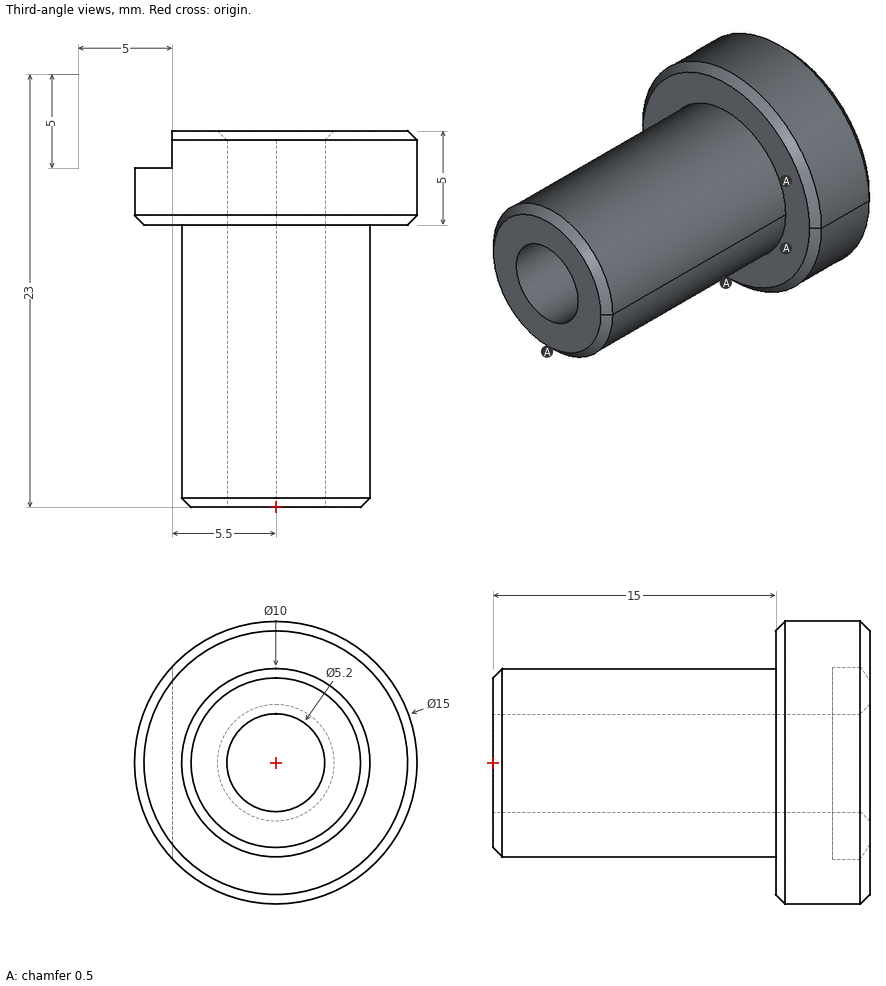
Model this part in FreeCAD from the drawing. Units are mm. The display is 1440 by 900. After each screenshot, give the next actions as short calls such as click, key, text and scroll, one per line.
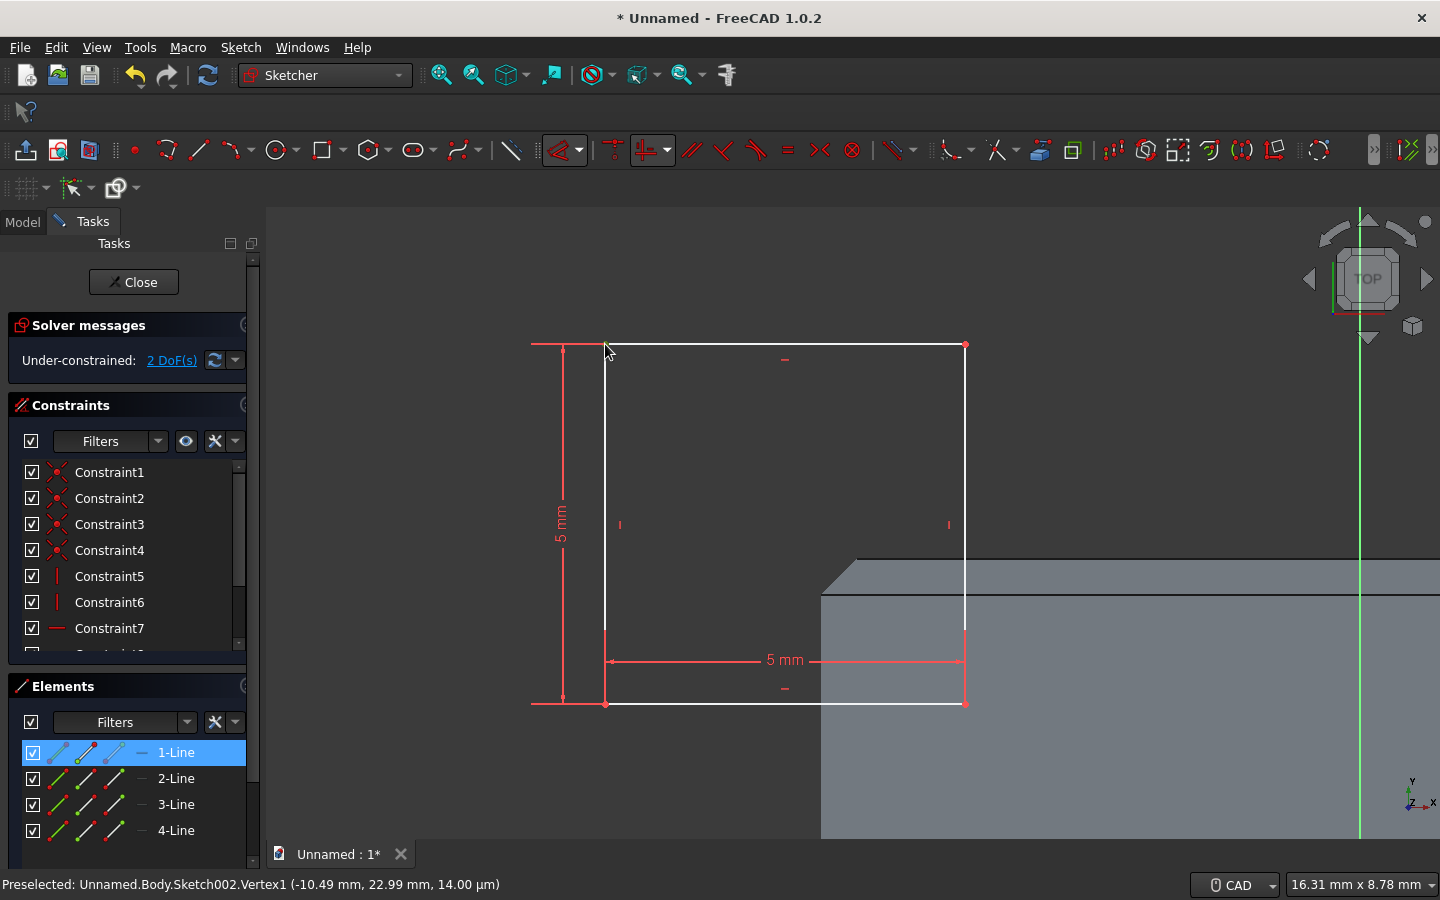
click(582, 150)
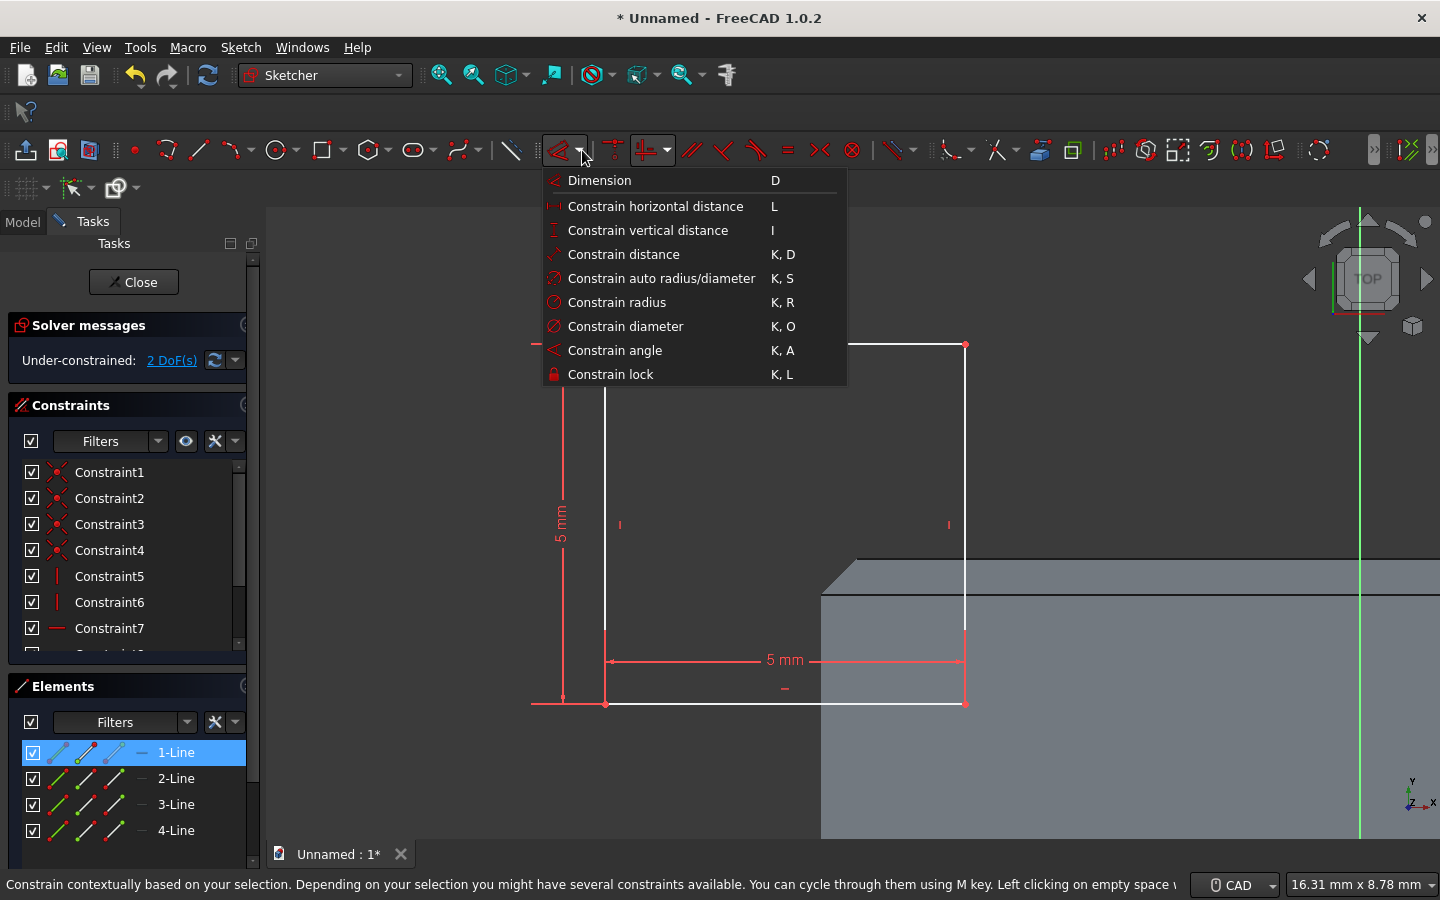
click(695, 230)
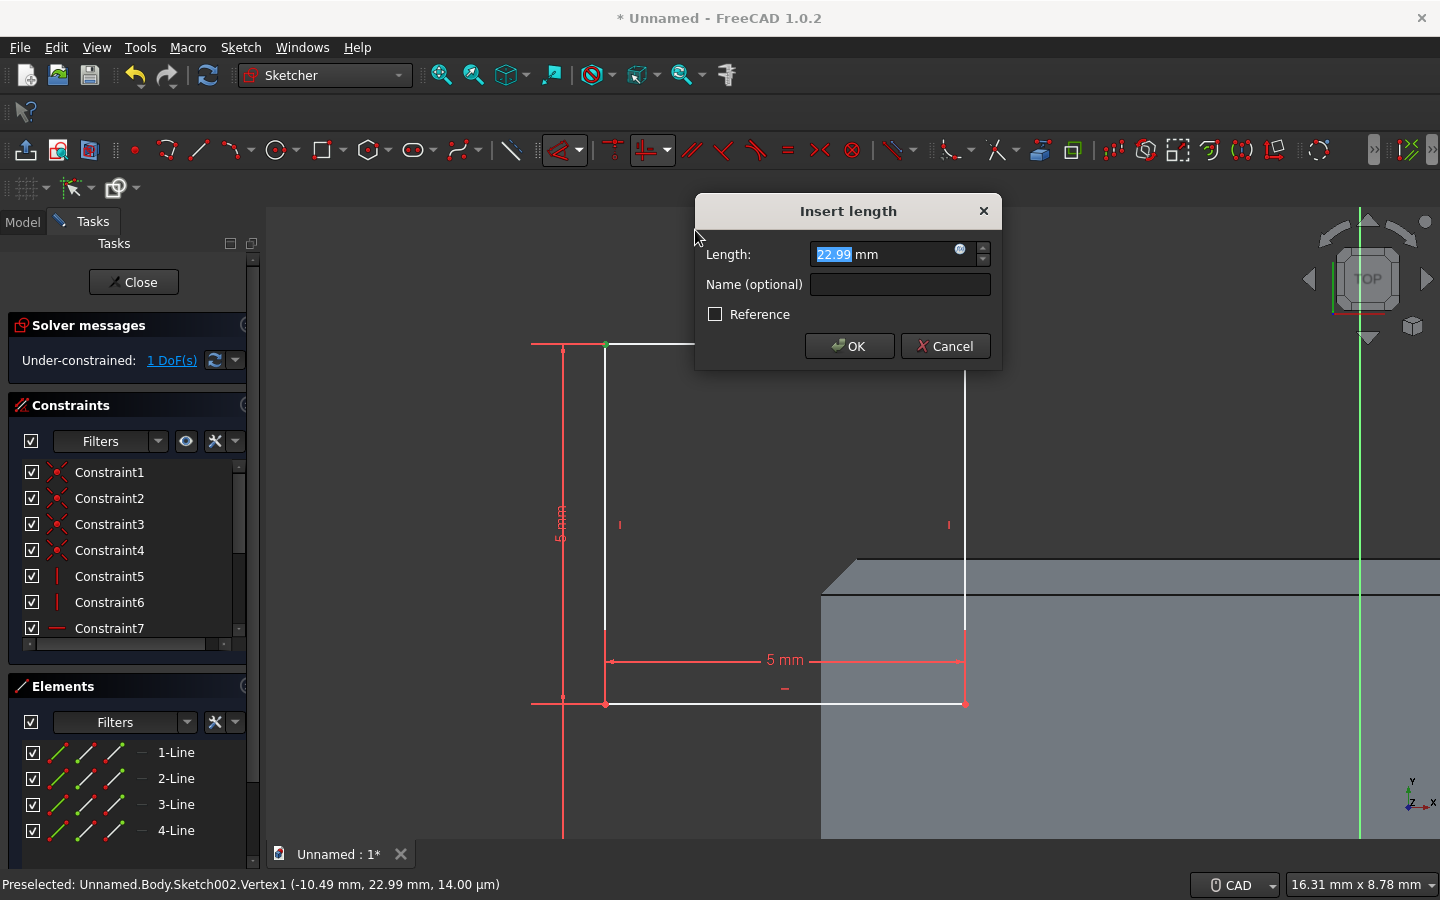
text(23)
key(Return)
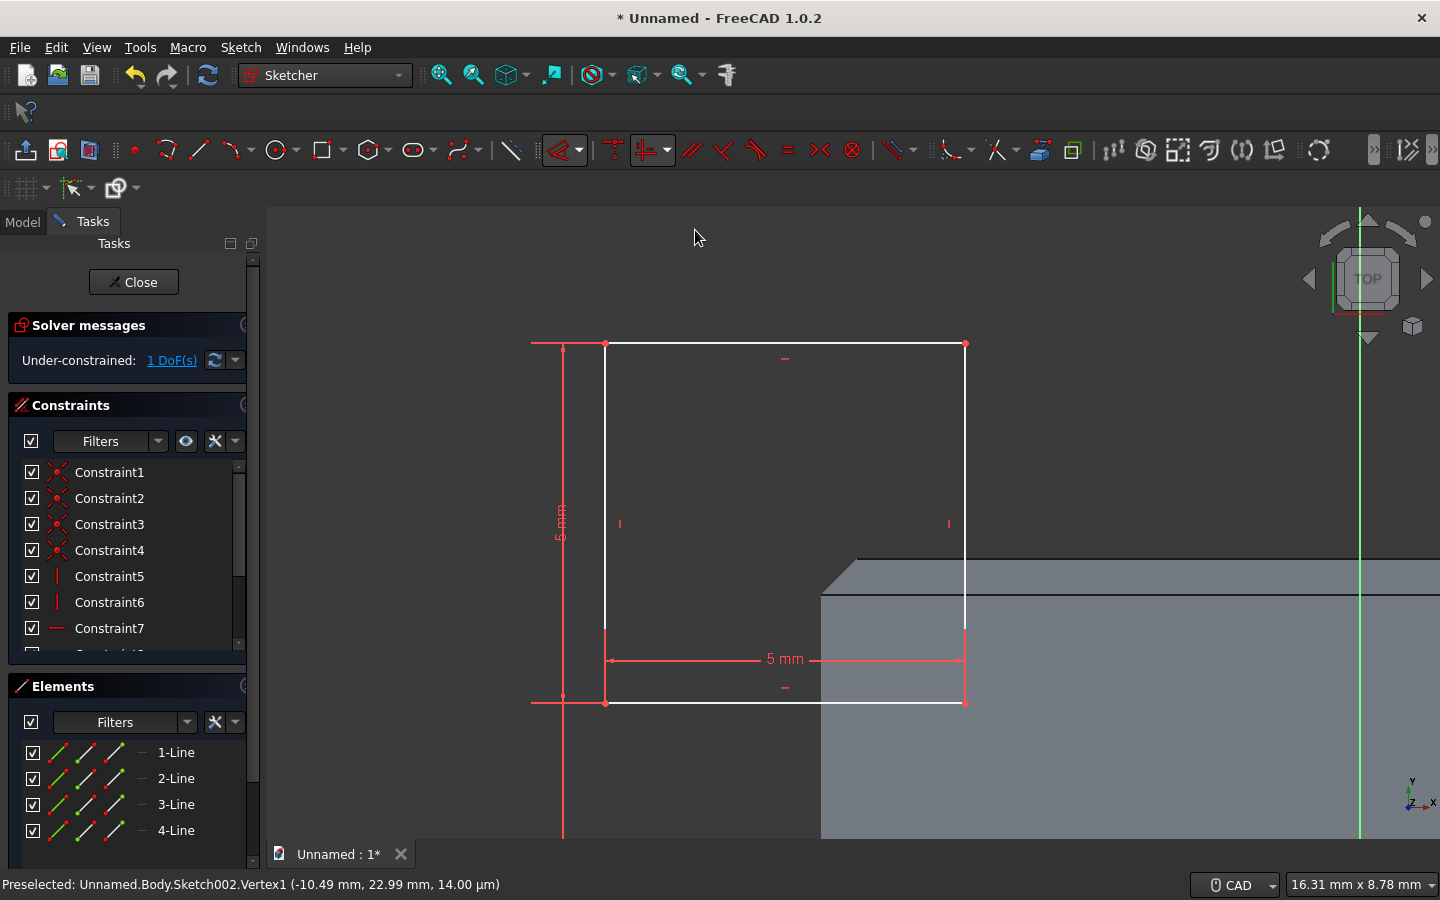
click(965, 703)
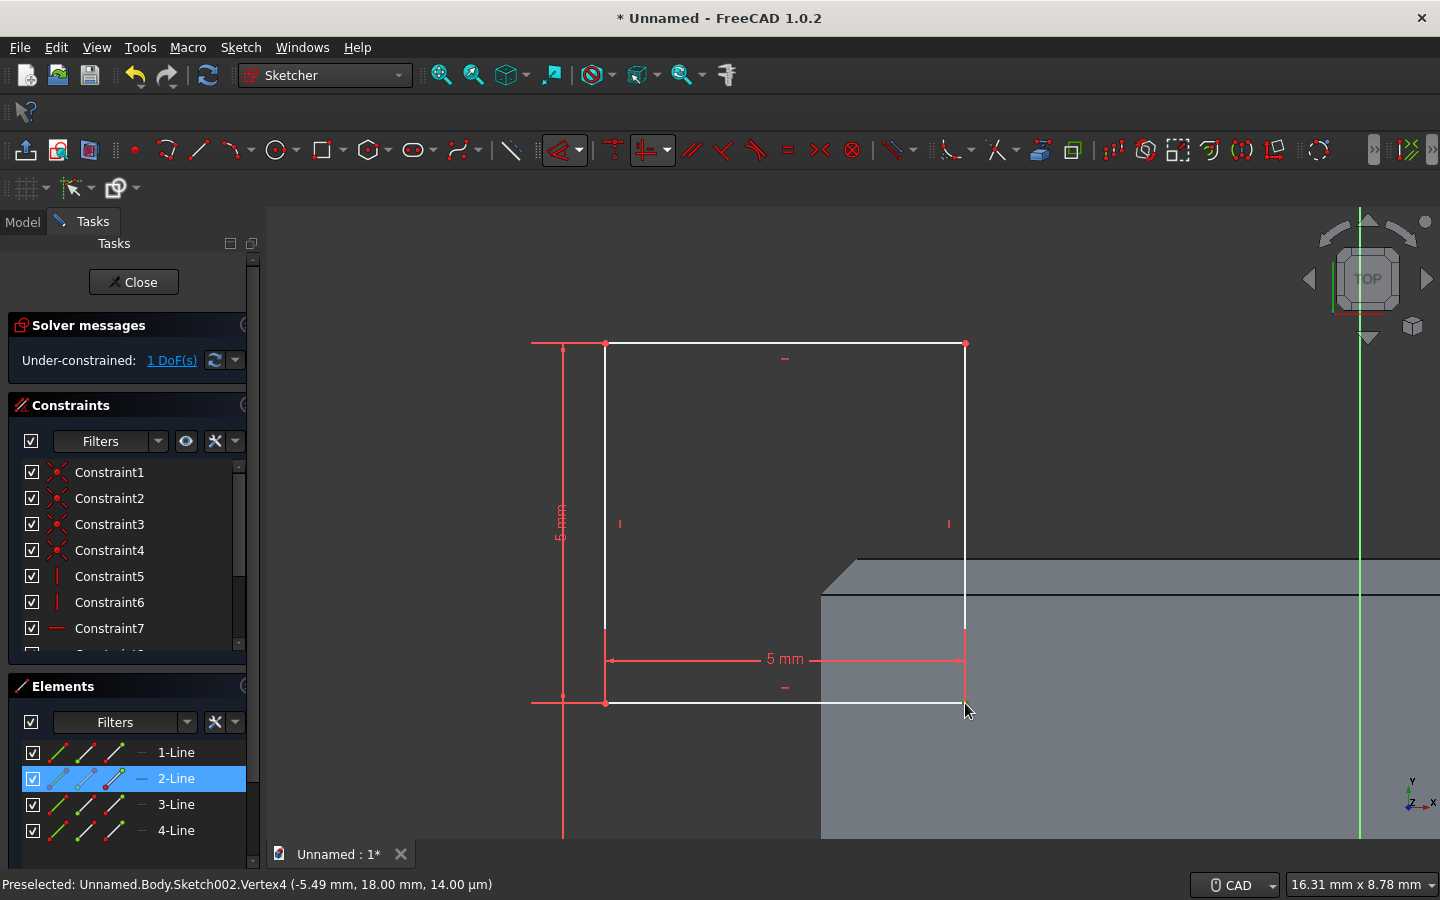
key(l)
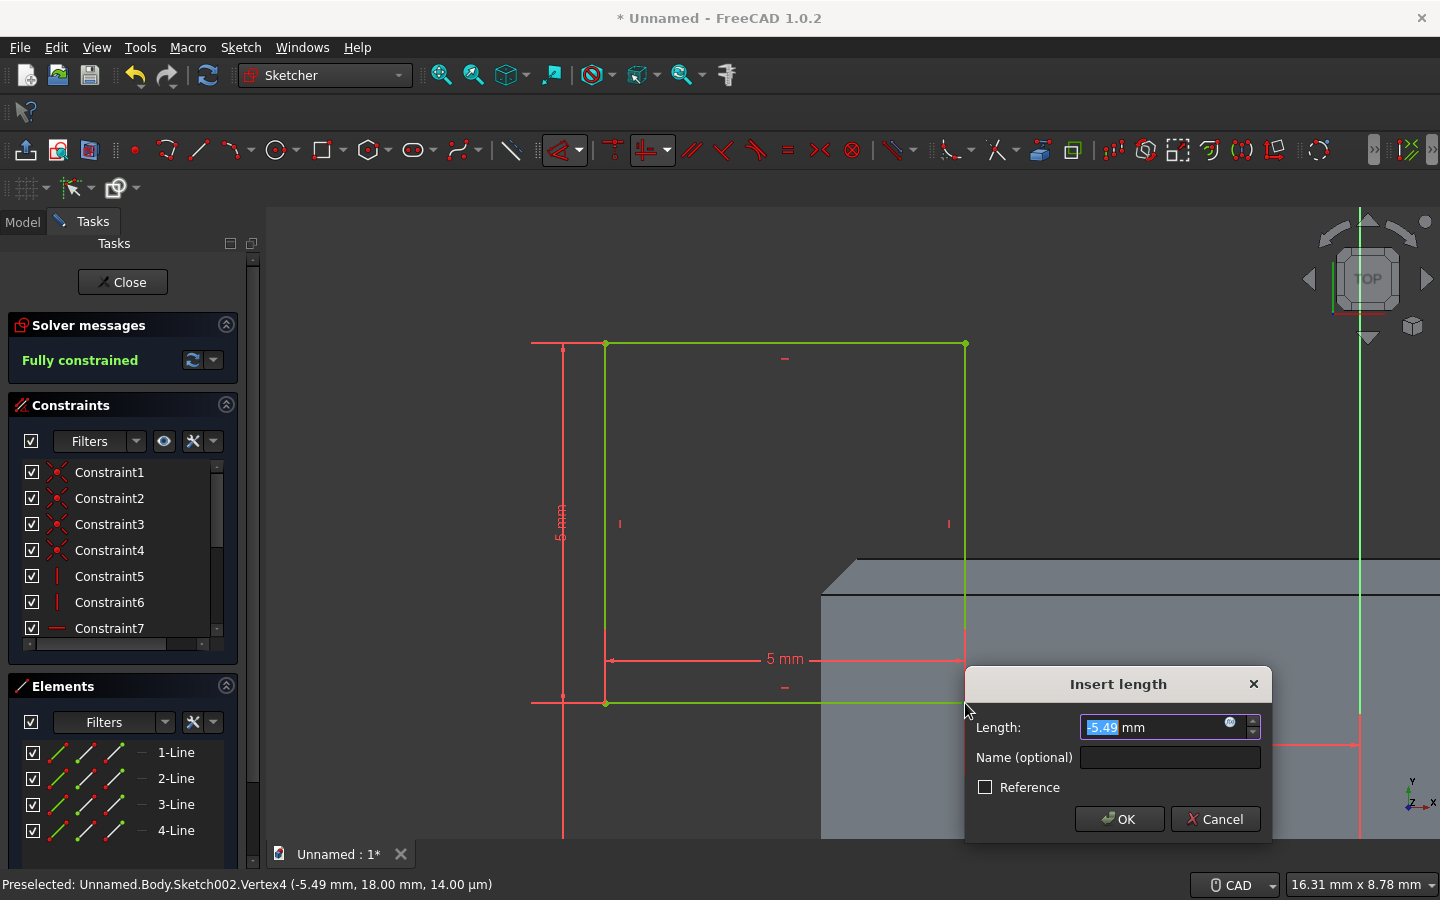
text(-5.5)
key(Return)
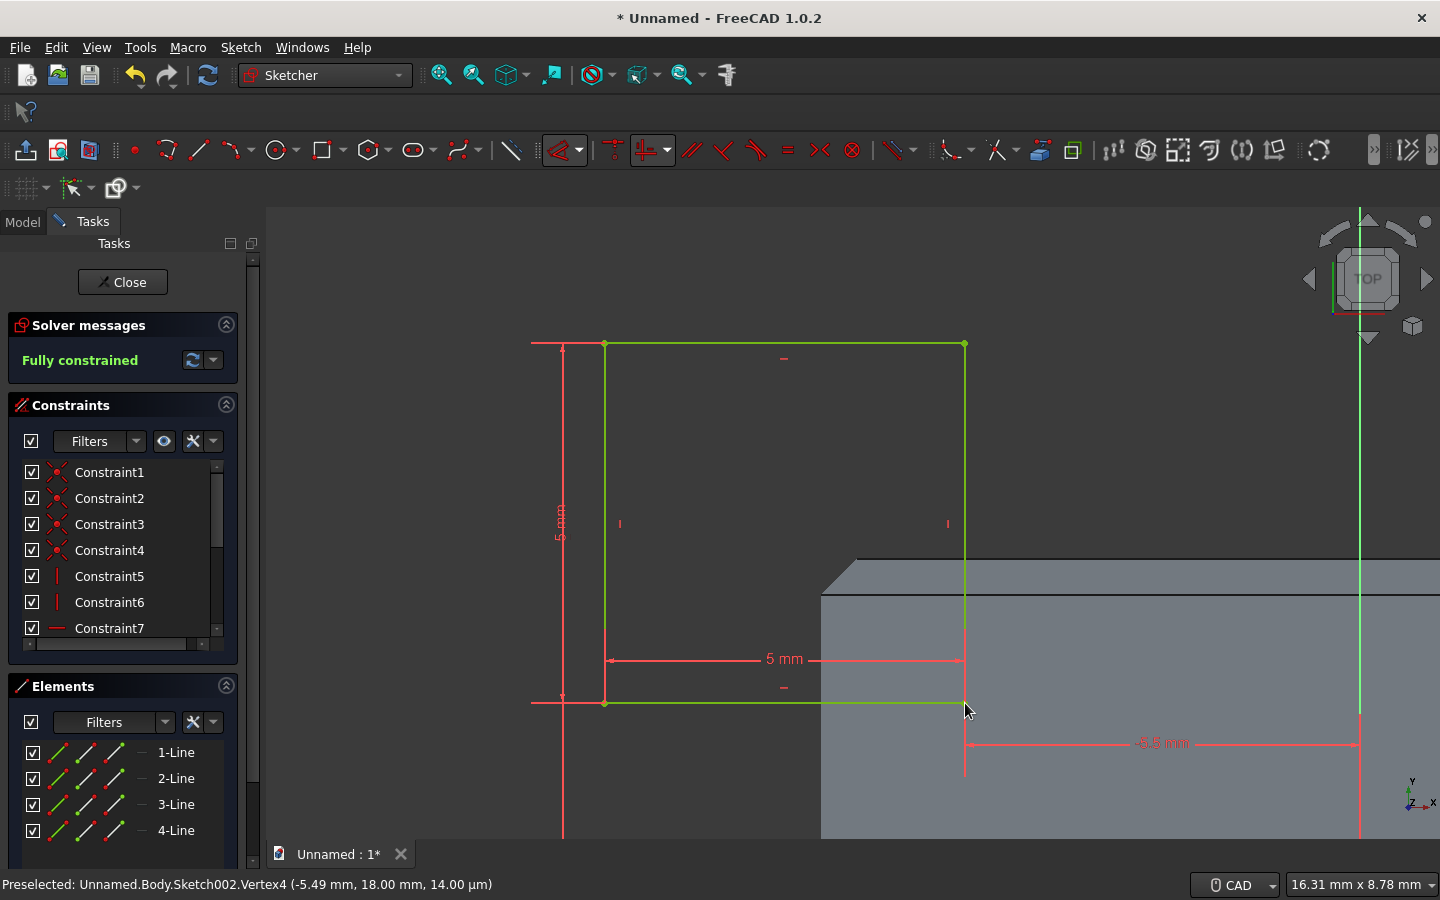
click(123, 282)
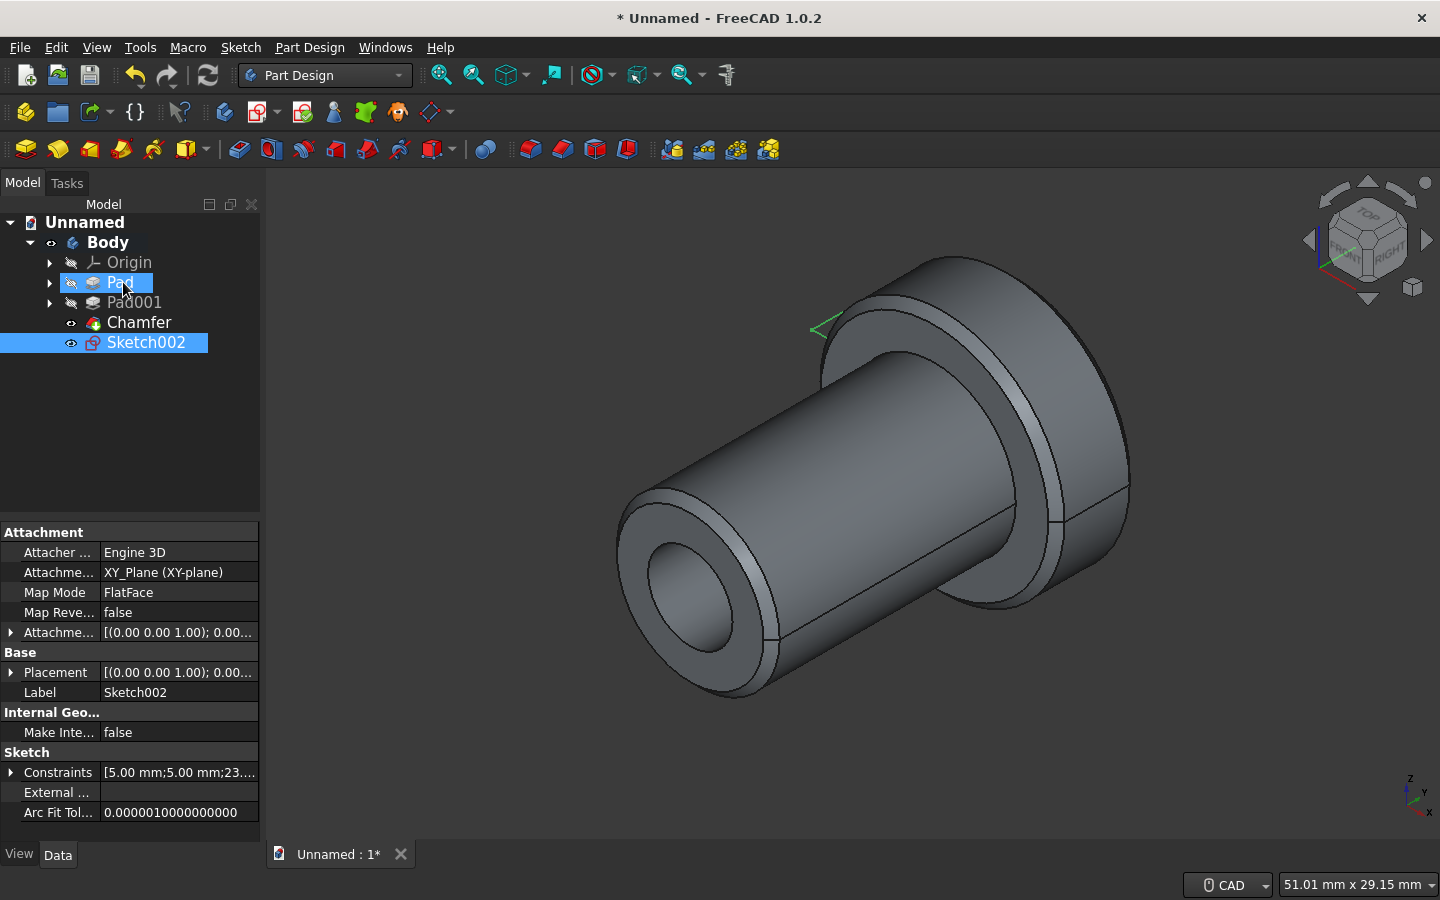
click(240, 150)